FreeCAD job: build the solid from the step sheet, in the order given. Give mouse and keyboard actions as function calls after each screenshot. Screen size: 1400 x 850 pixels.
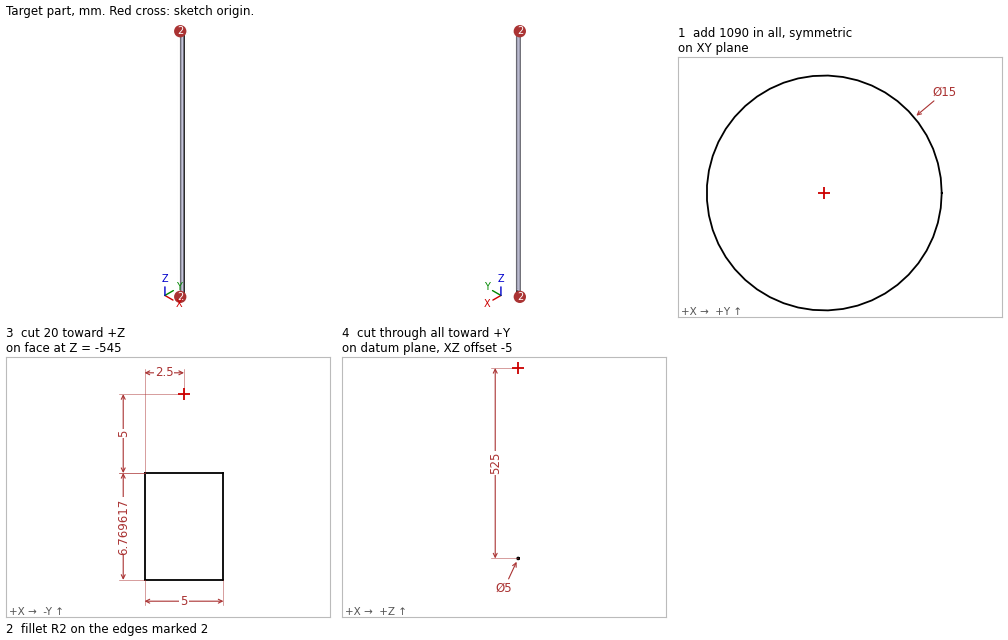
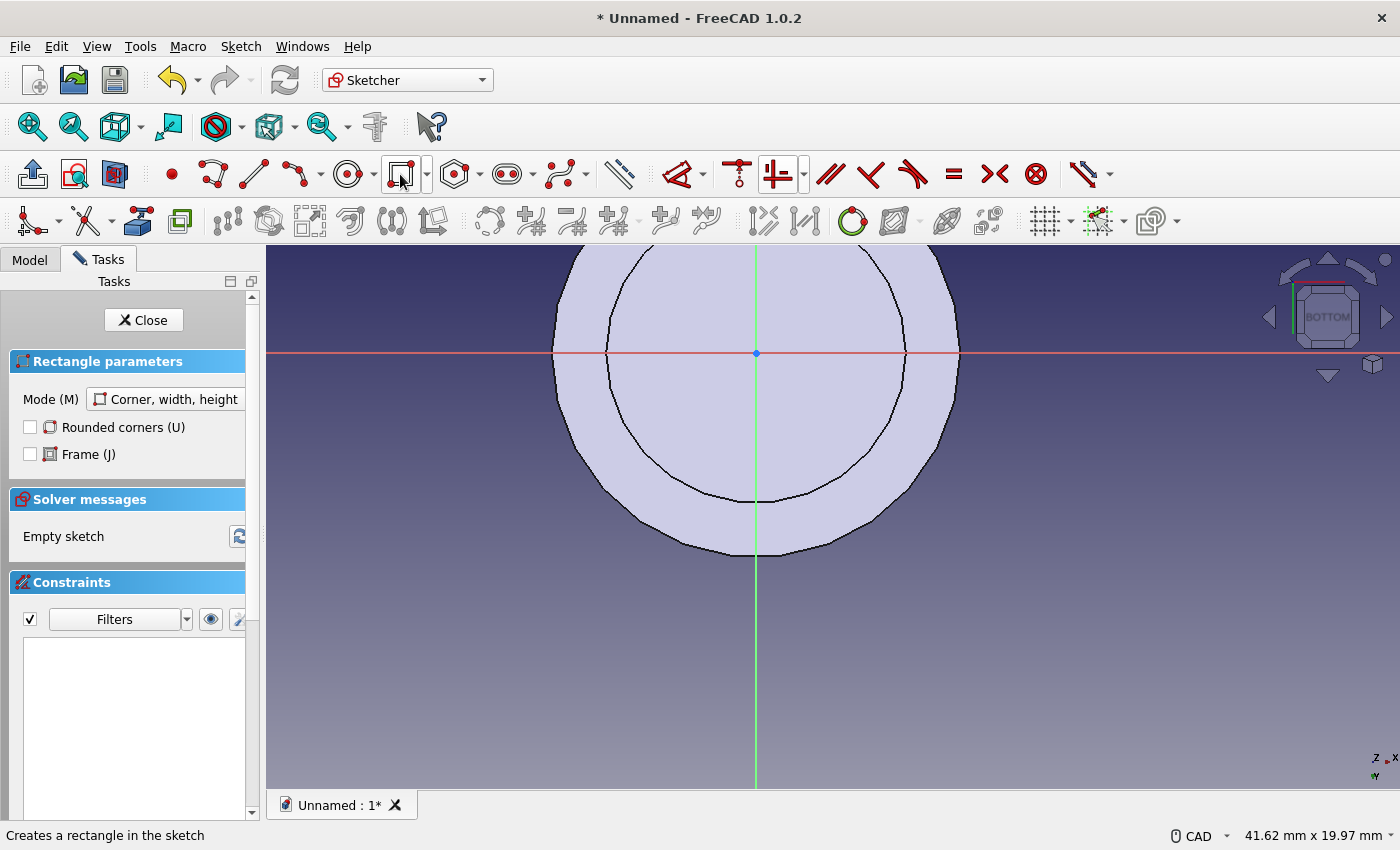
click(688, 489)
click(824, 674)
key(Escape)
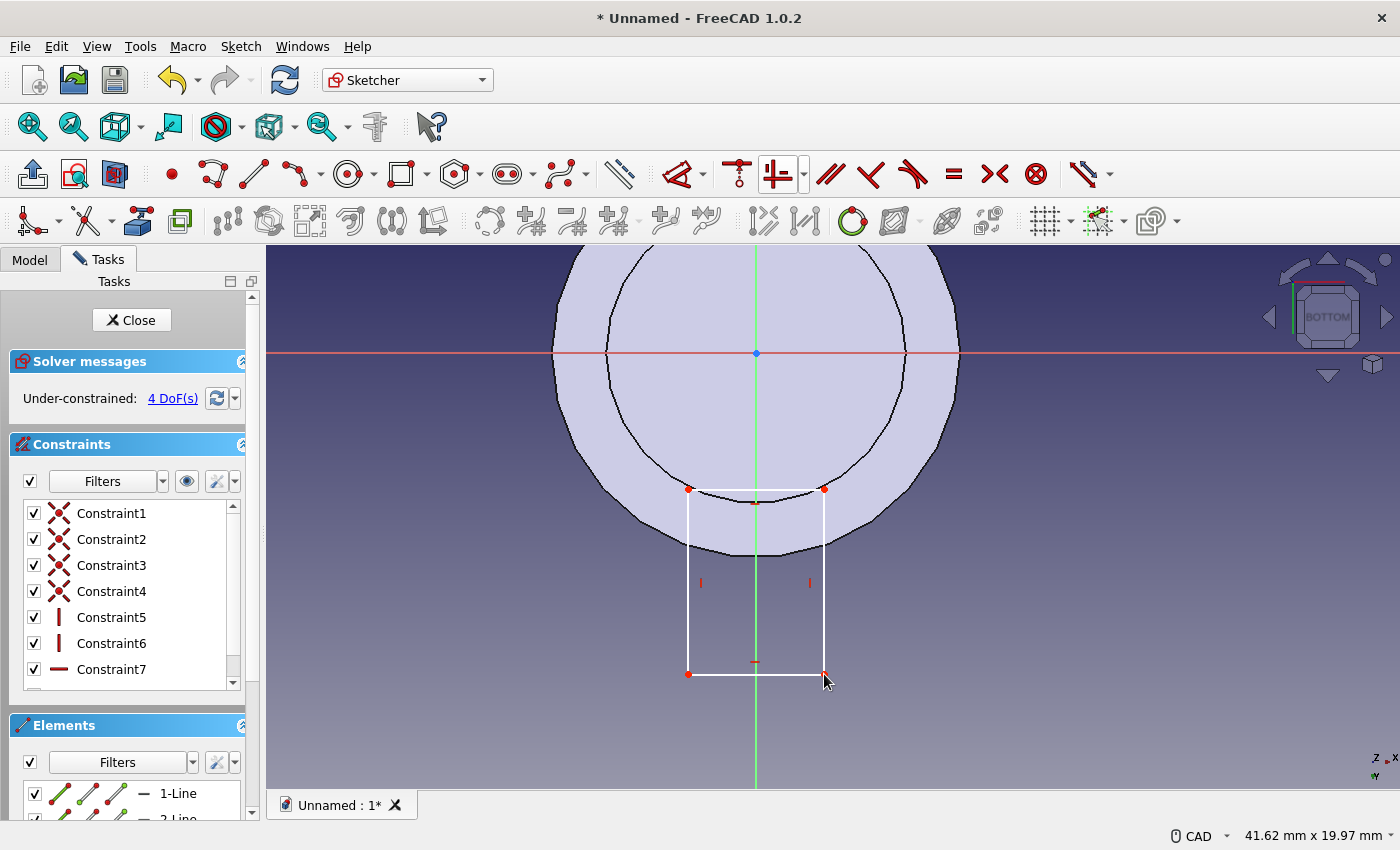
click(676, 174)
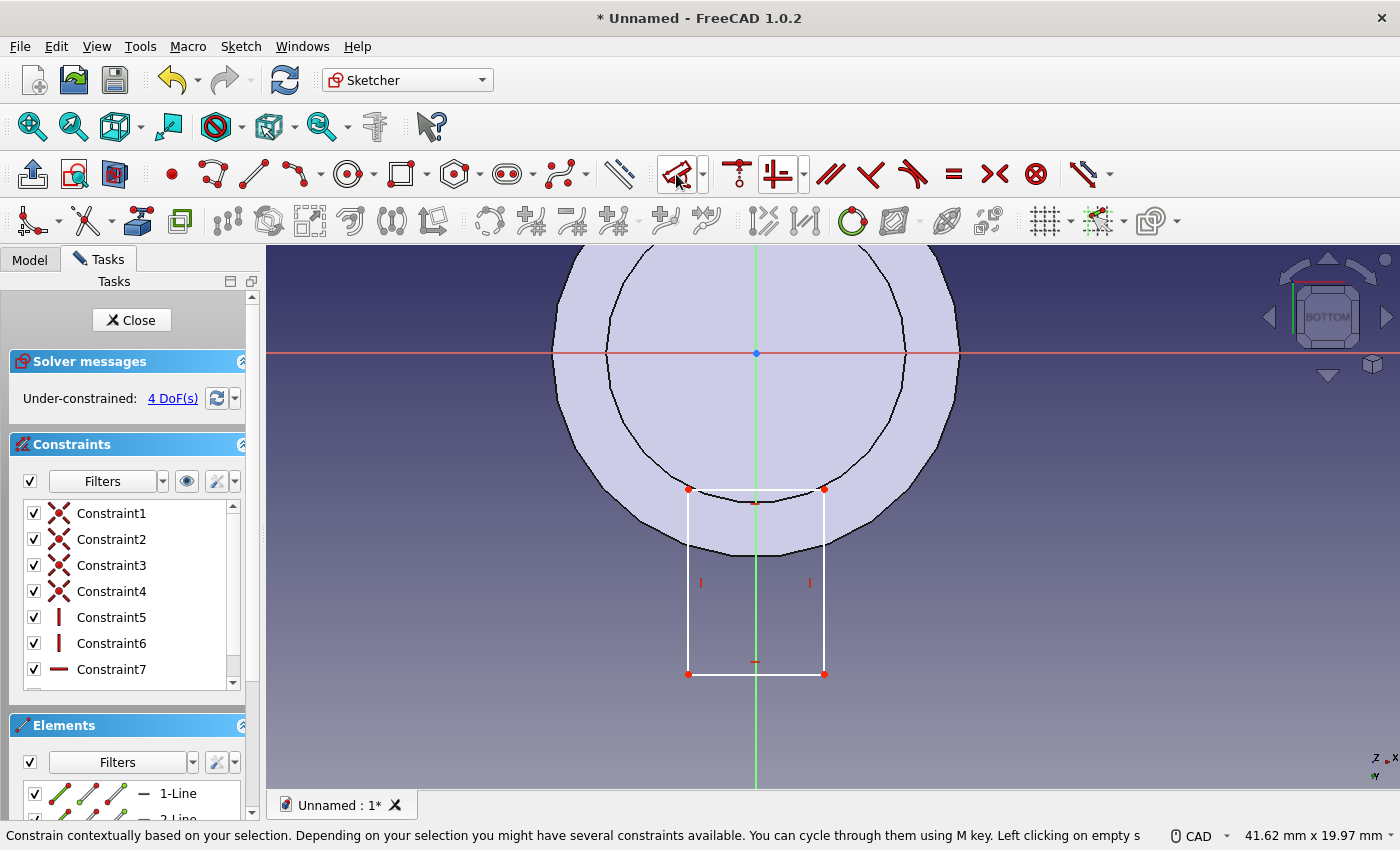
click(729, 675)
click(725, 709)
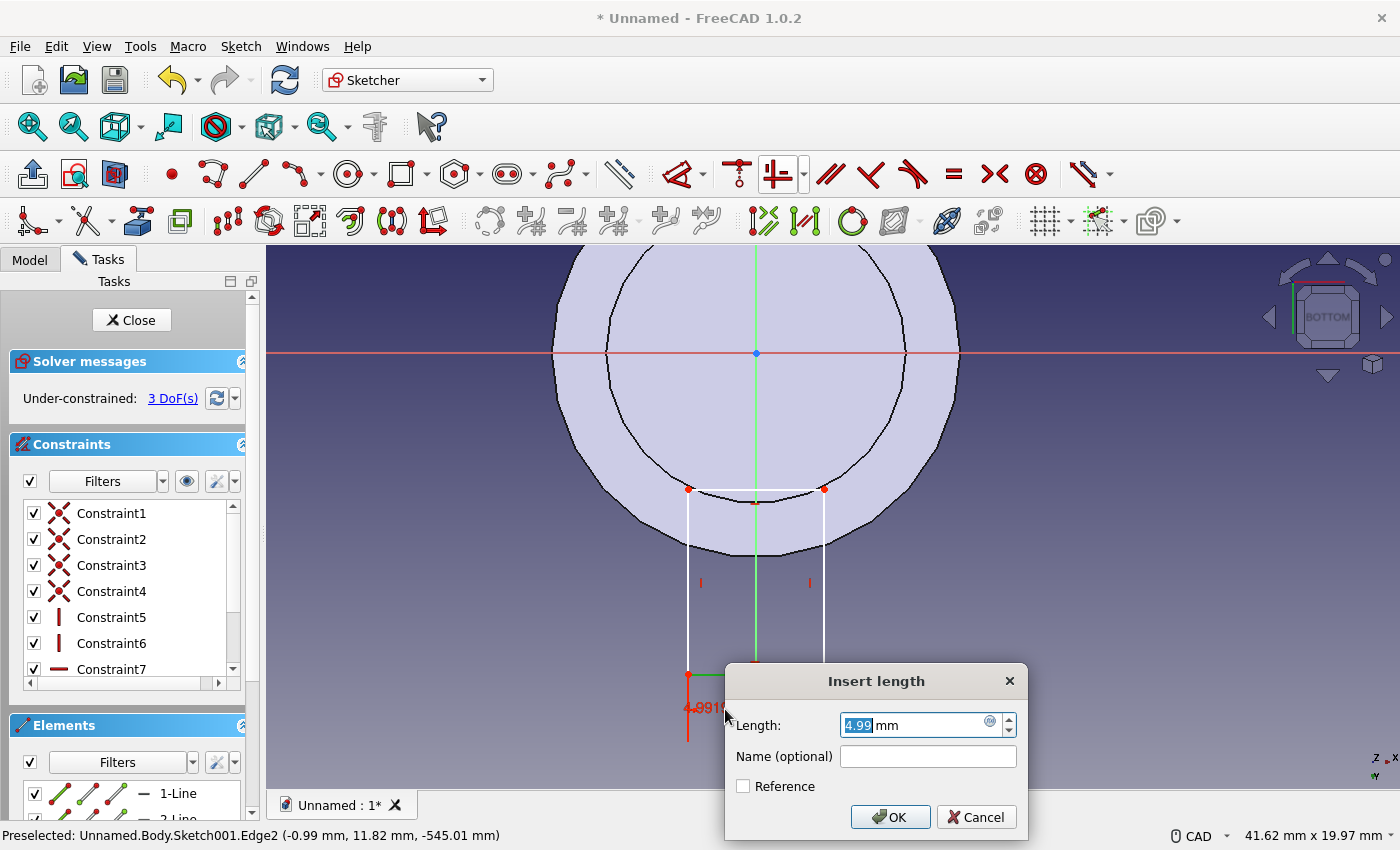
text(5)
key(Return)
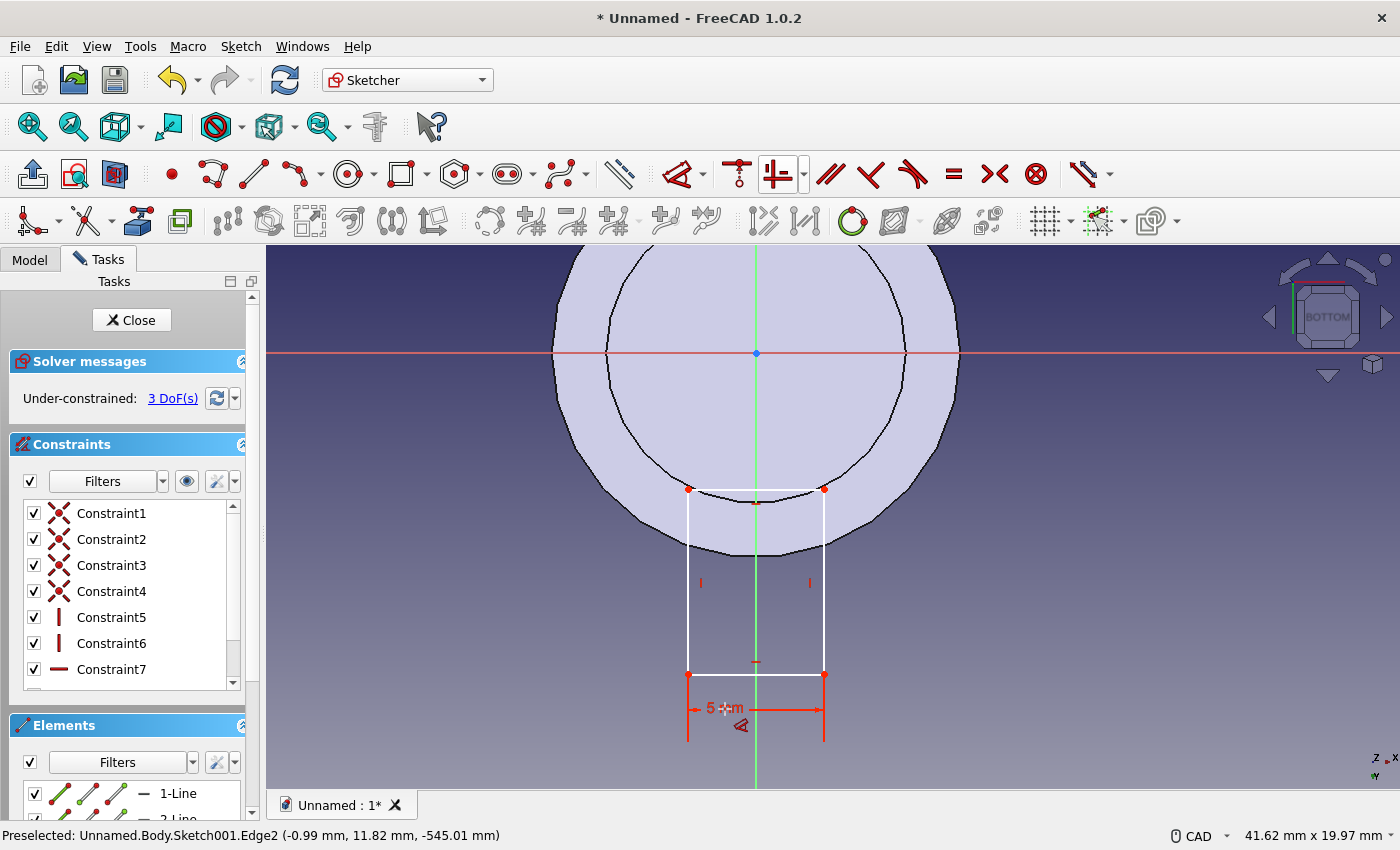
click(688, 490)
click(654, 422)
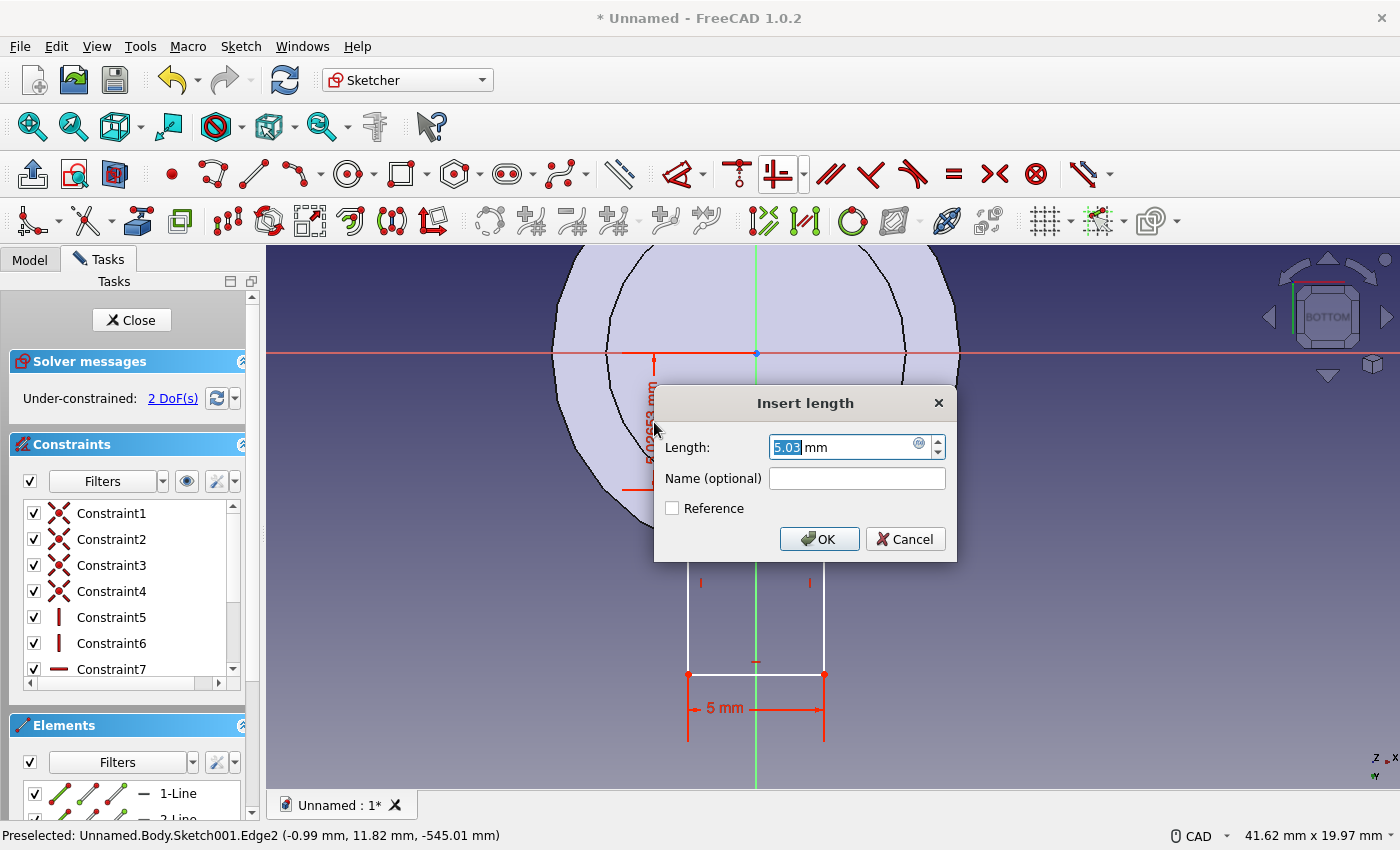
text(5)
key(Return)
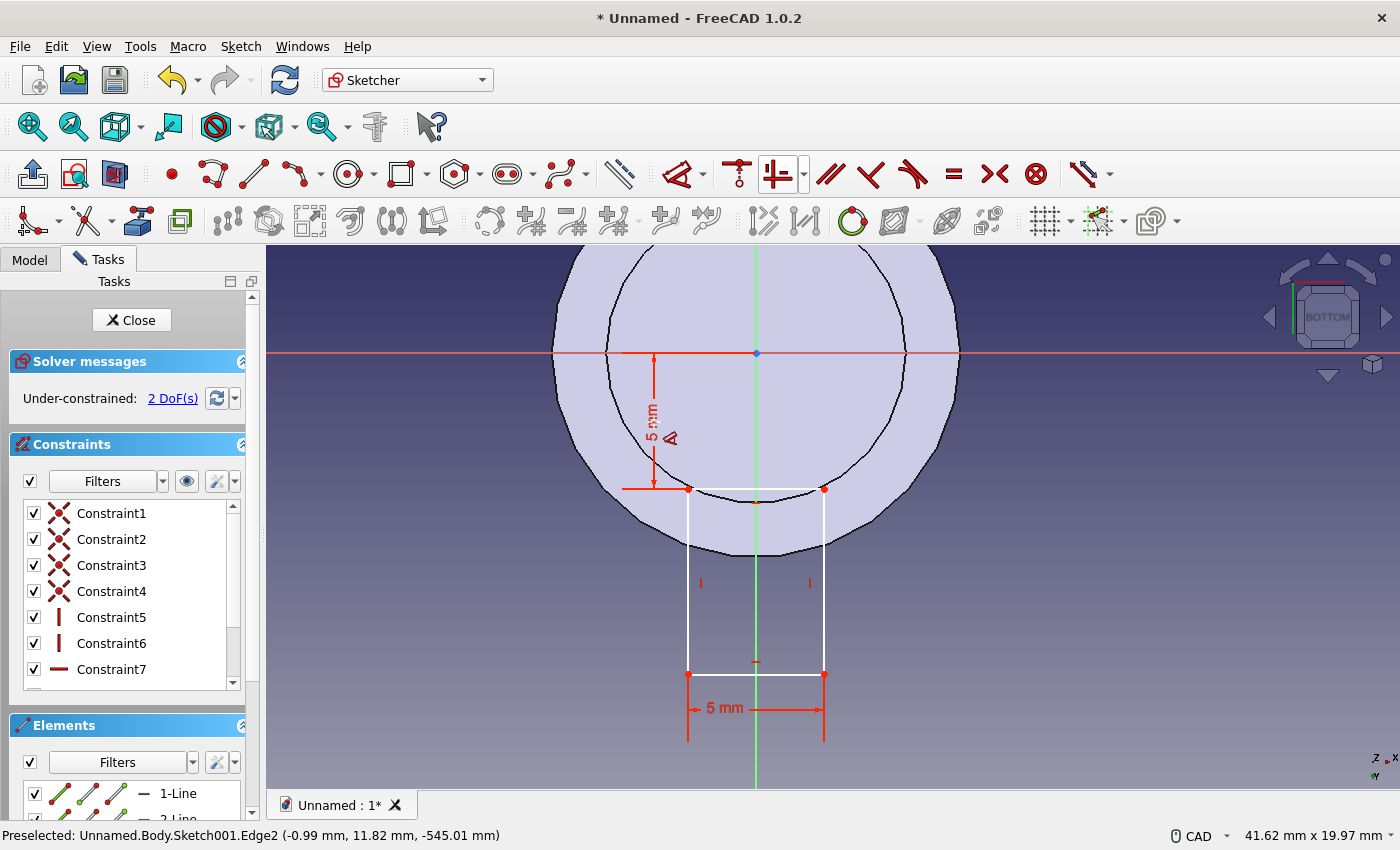
click(688, 489)
click(722, 319)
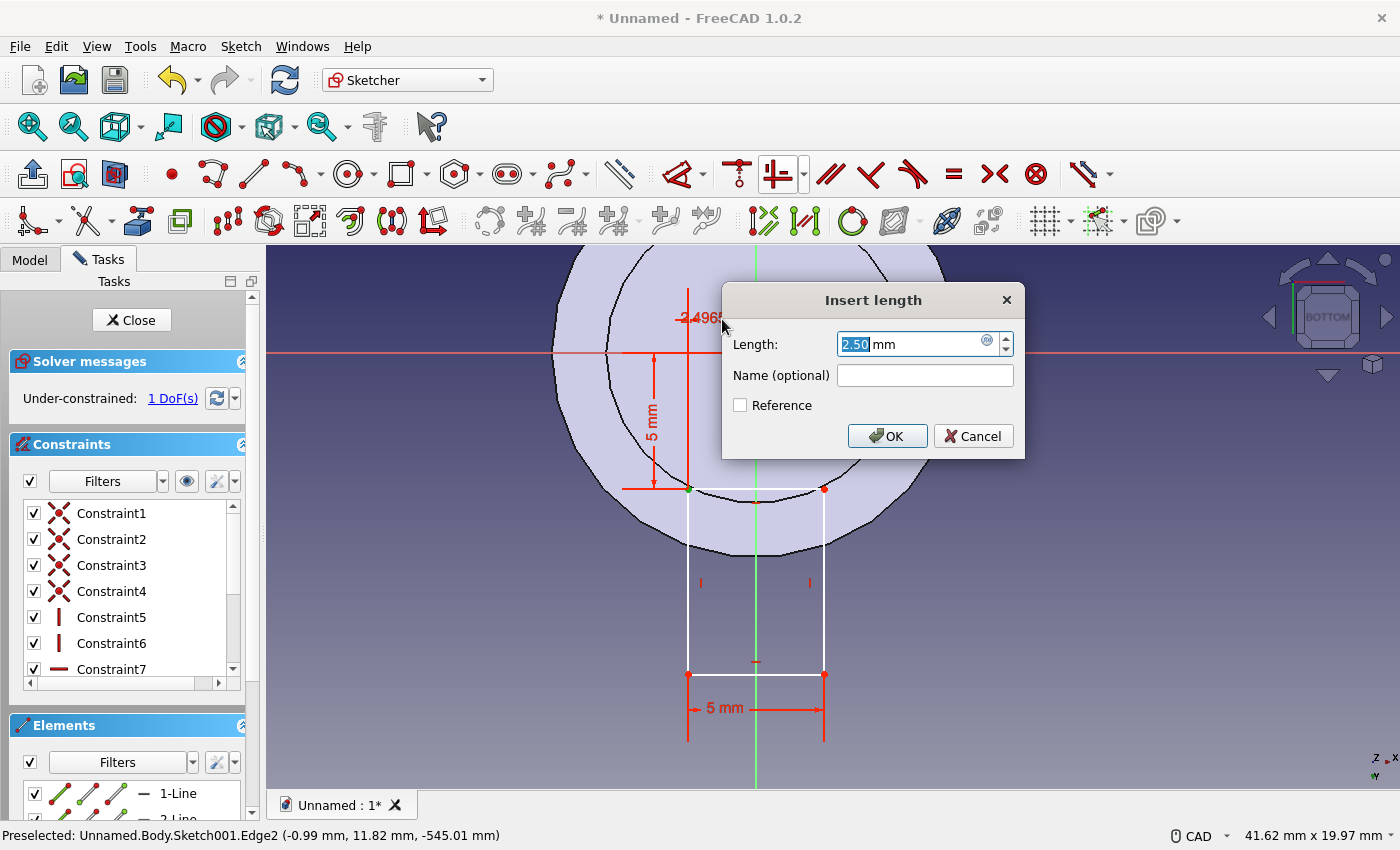
text(2.5)
key(Return)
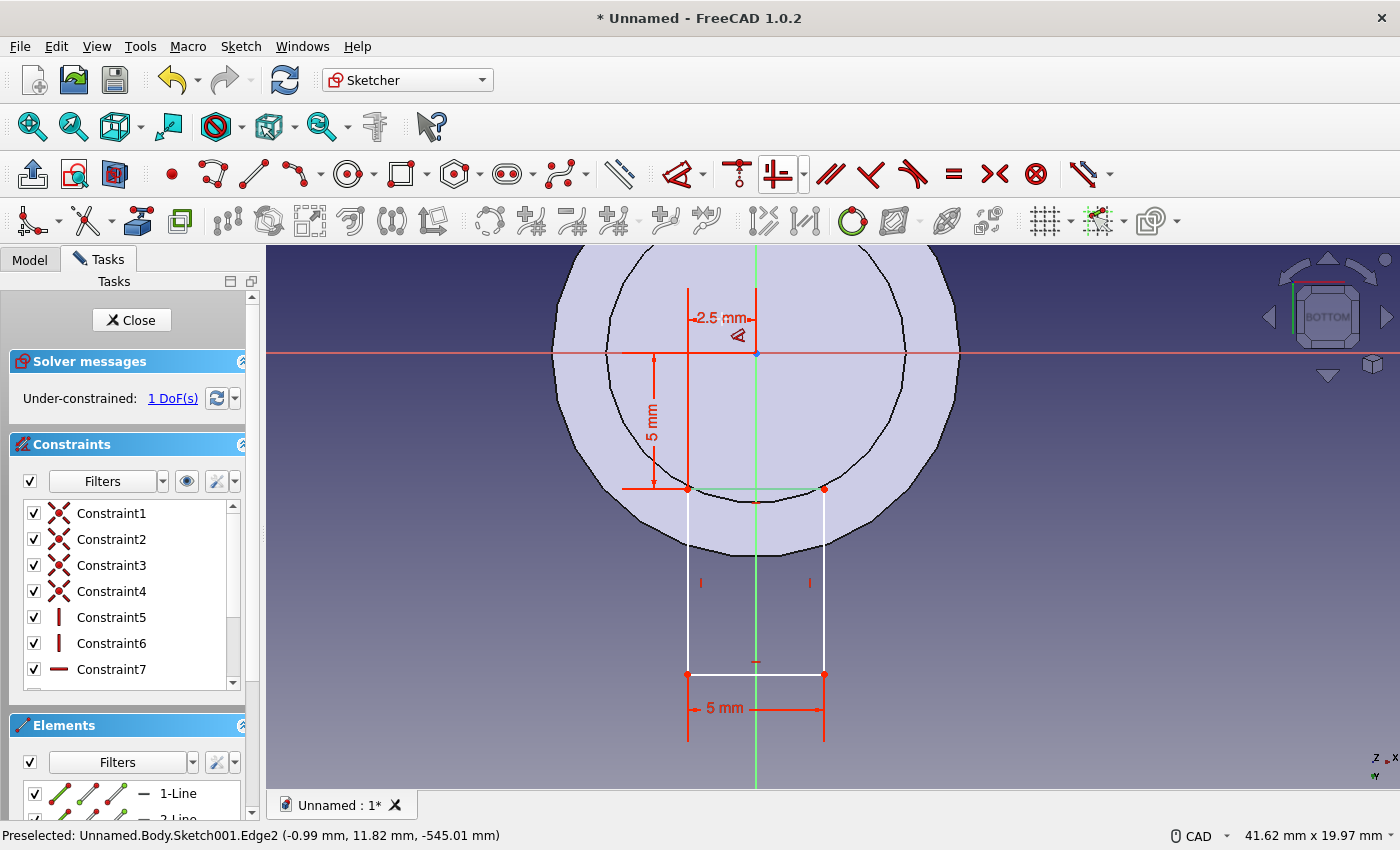
click(688, 545)
click(654, 582)